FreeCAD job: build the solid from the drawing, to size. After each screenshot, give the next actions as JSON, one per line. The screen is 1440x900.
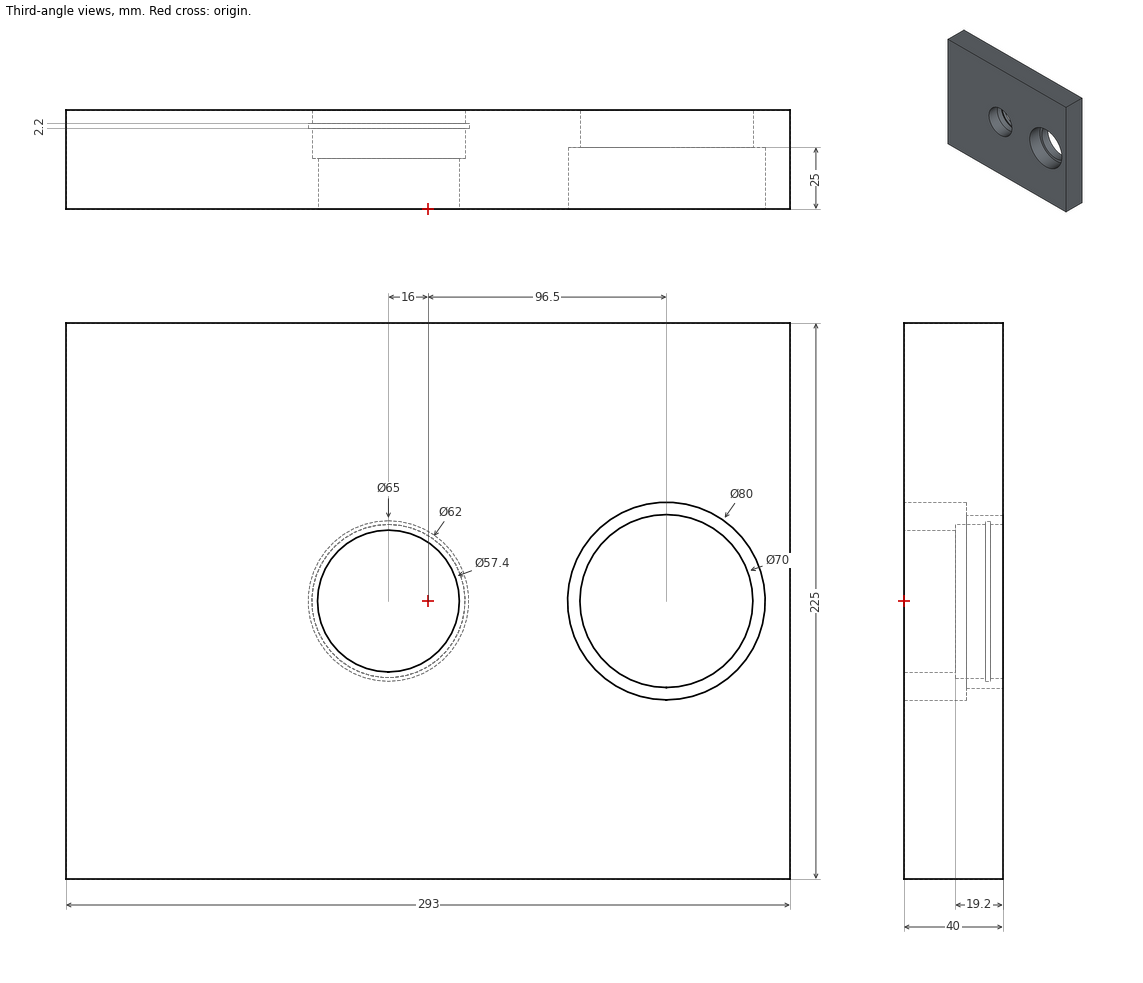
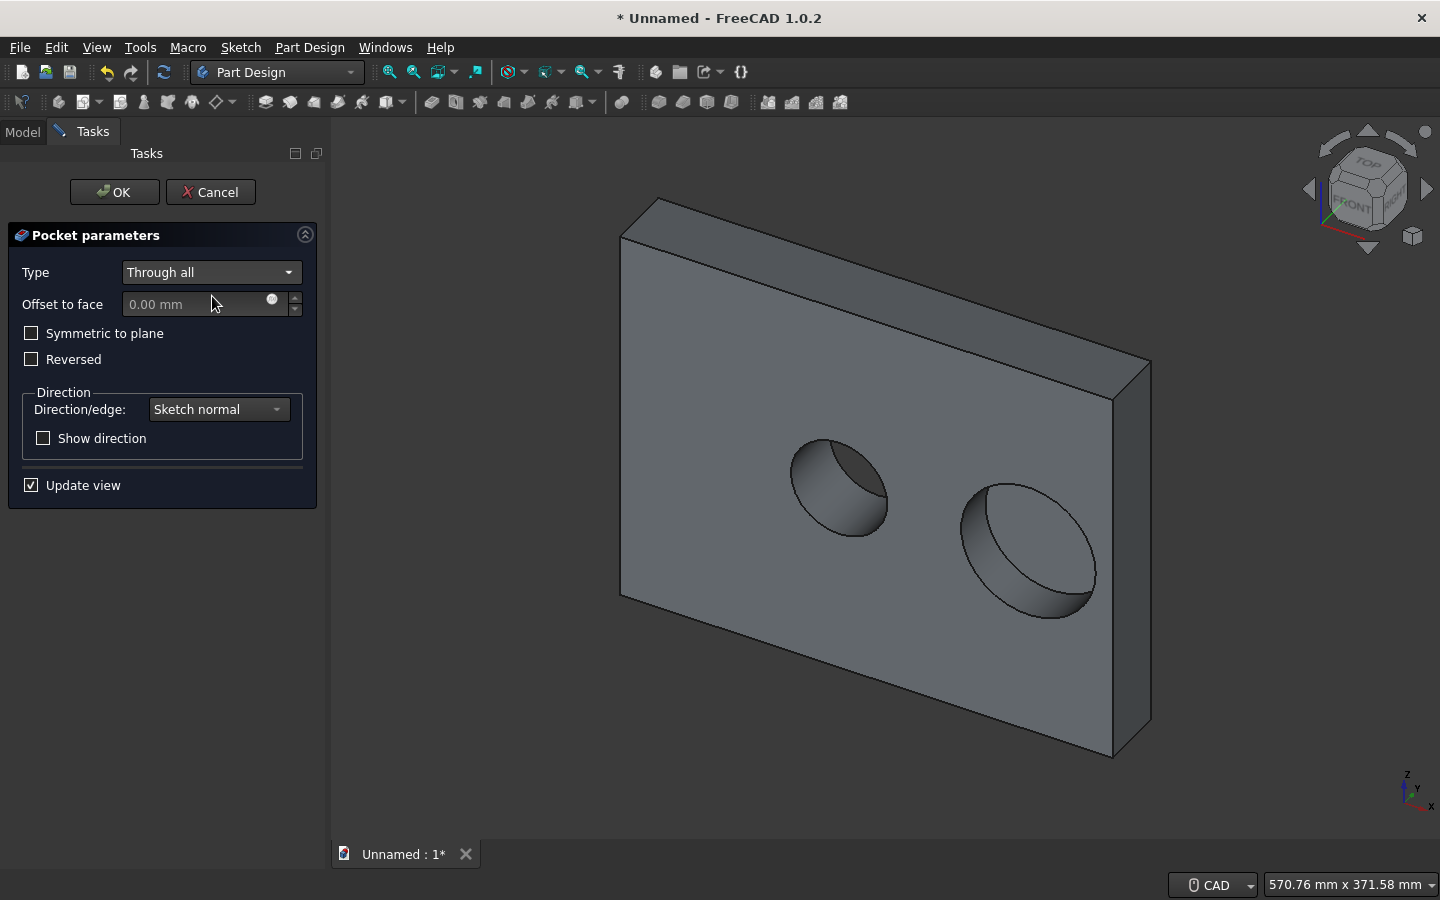
{"action": "left_click", "coordinate": [115, 192]}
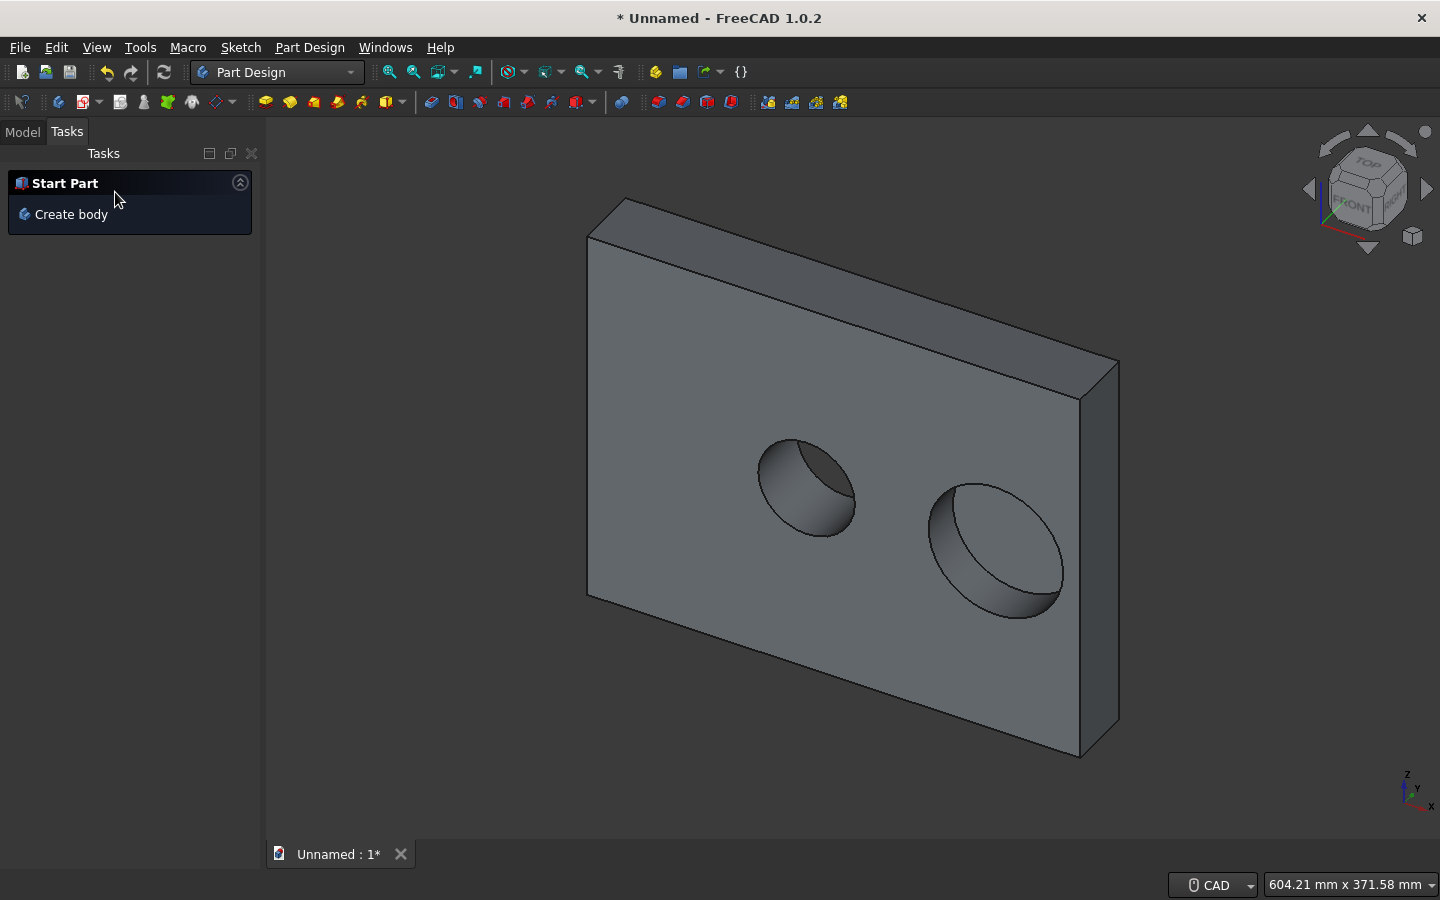
{"action": "left_click", "coordinate": [84, 102]}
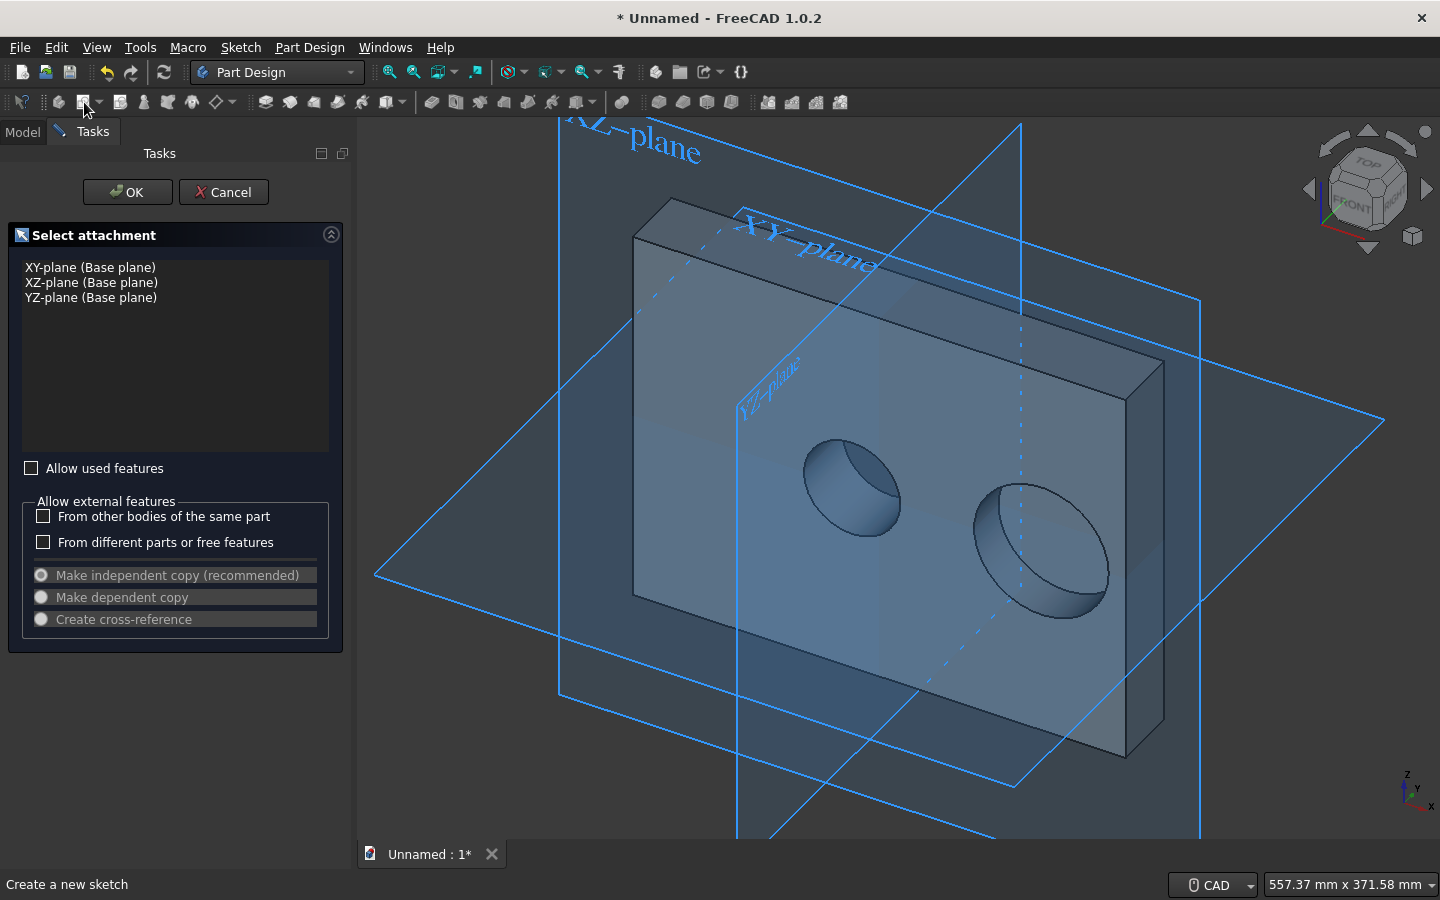
{"action": "left_click", "coordinate": [82, 282]}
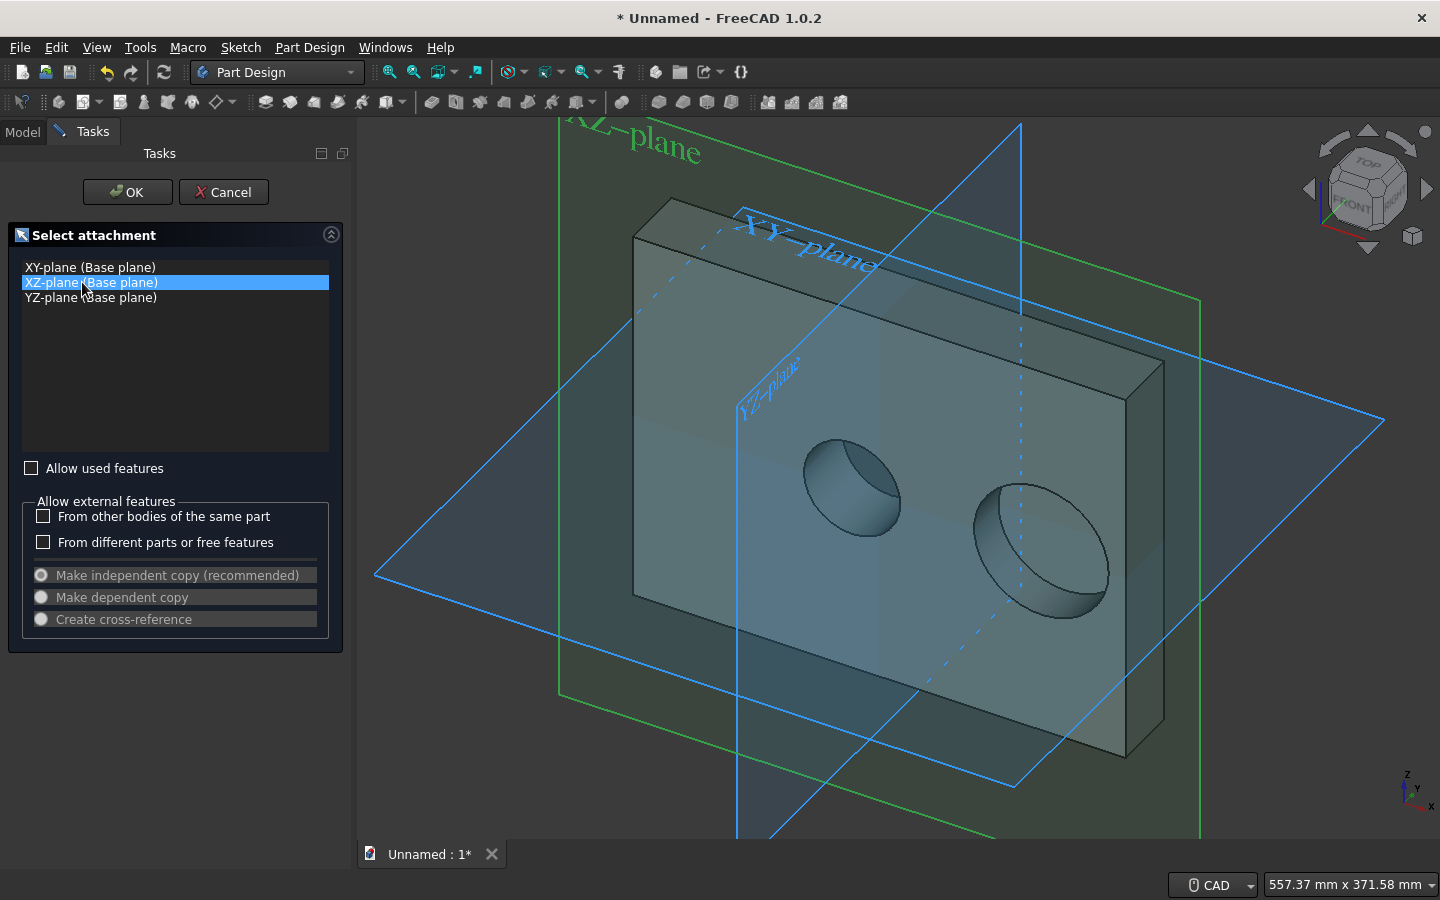
{"action": "left_click", "coordinate": [128, 192]}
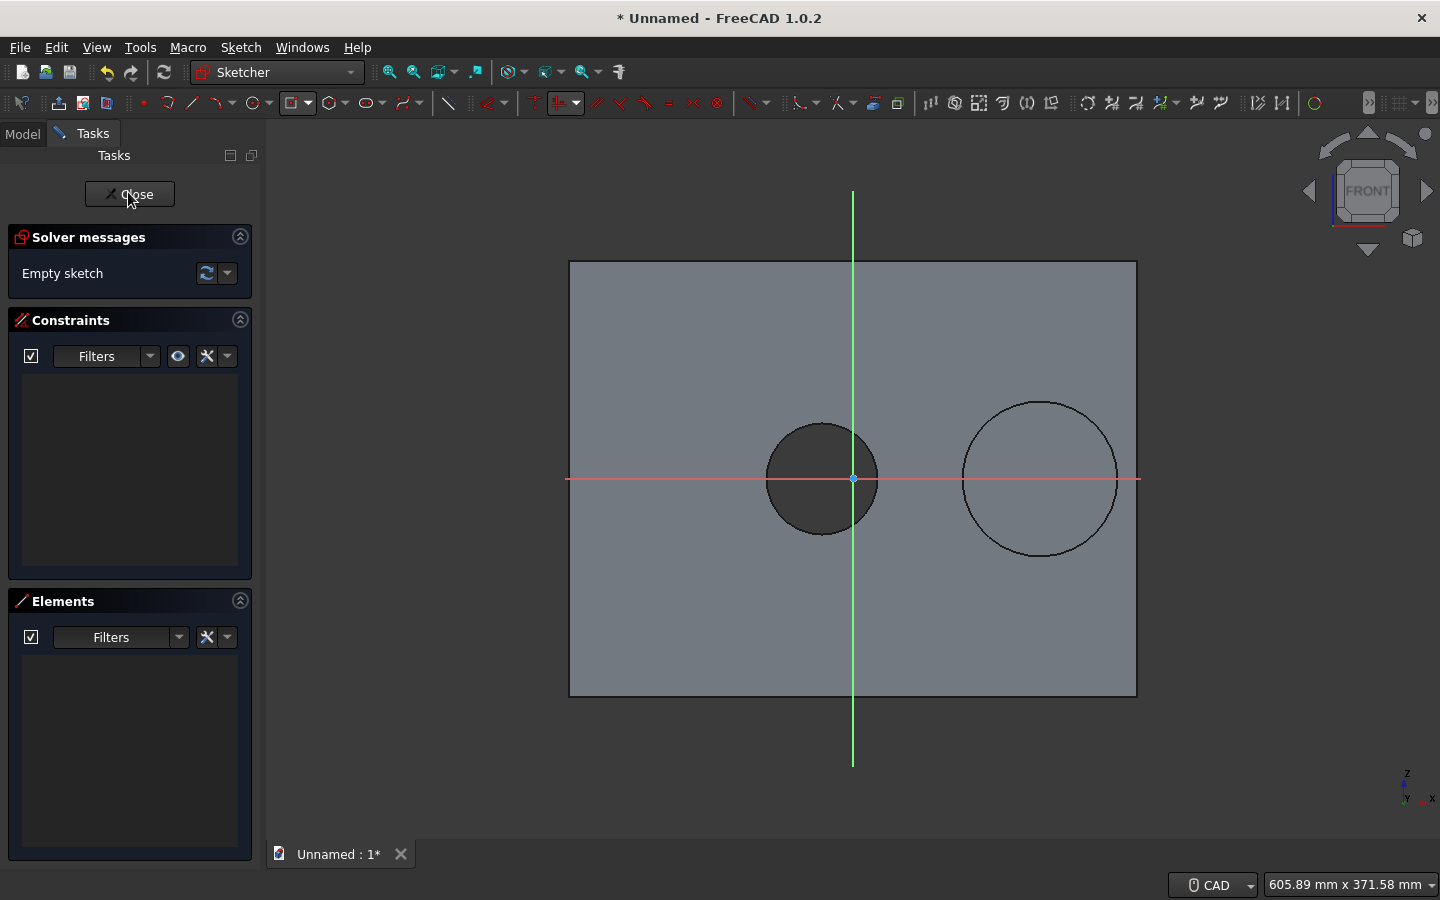
{"action": "scroll", "coordinate": [1094, 479], "scroll_direction": "up", "scroll_amount": 5}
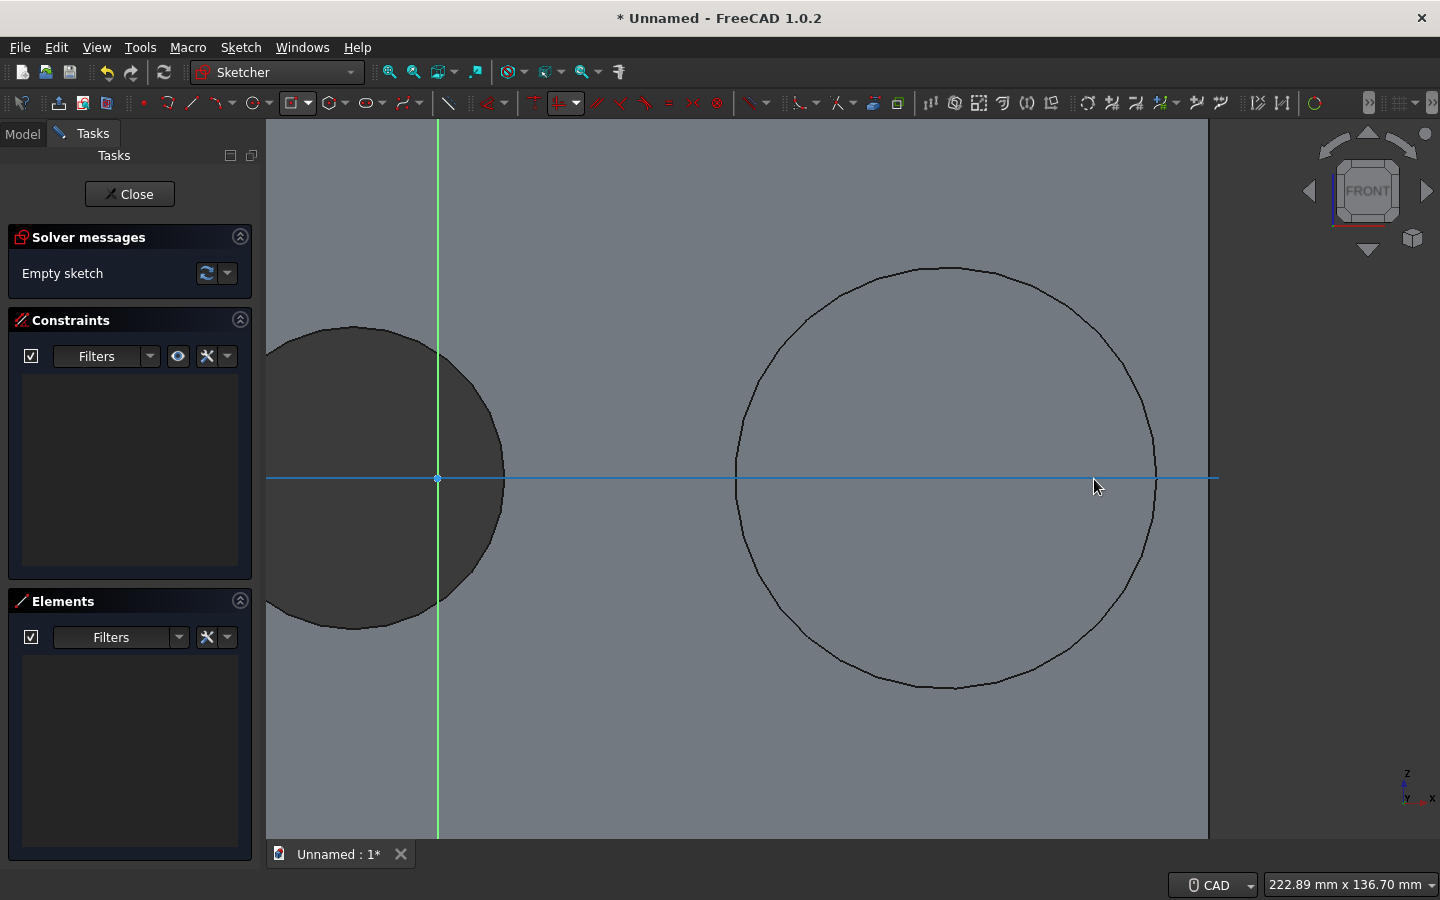
{"action": "left_click", "coordinate": [254, 104]}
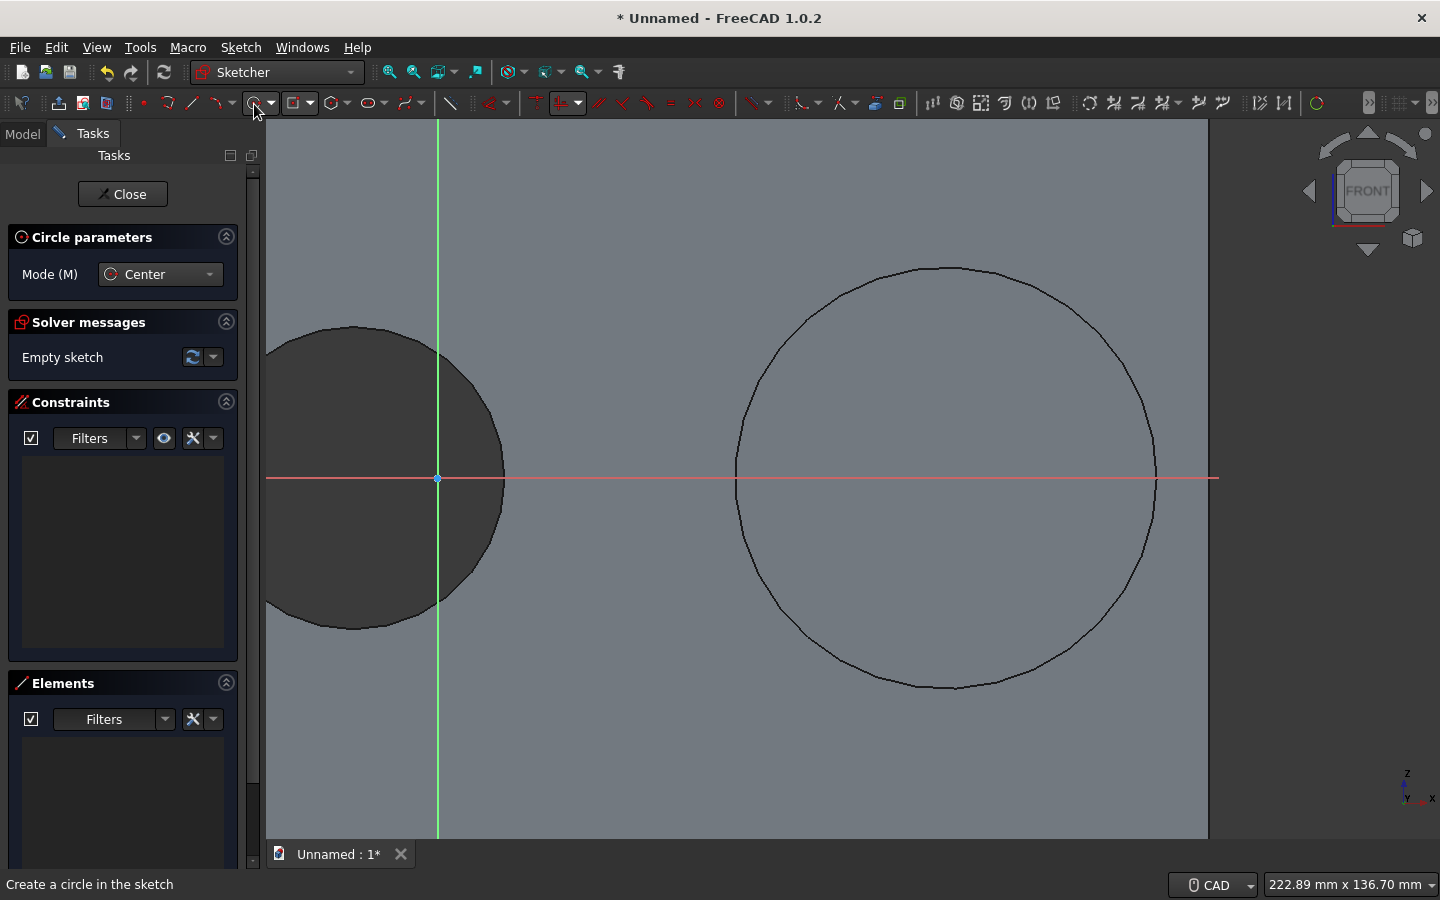
{"action": "left_click", "coordinate": [946, 478]}
{"action": "mouse_move", "coordinate": [1076, 348]}